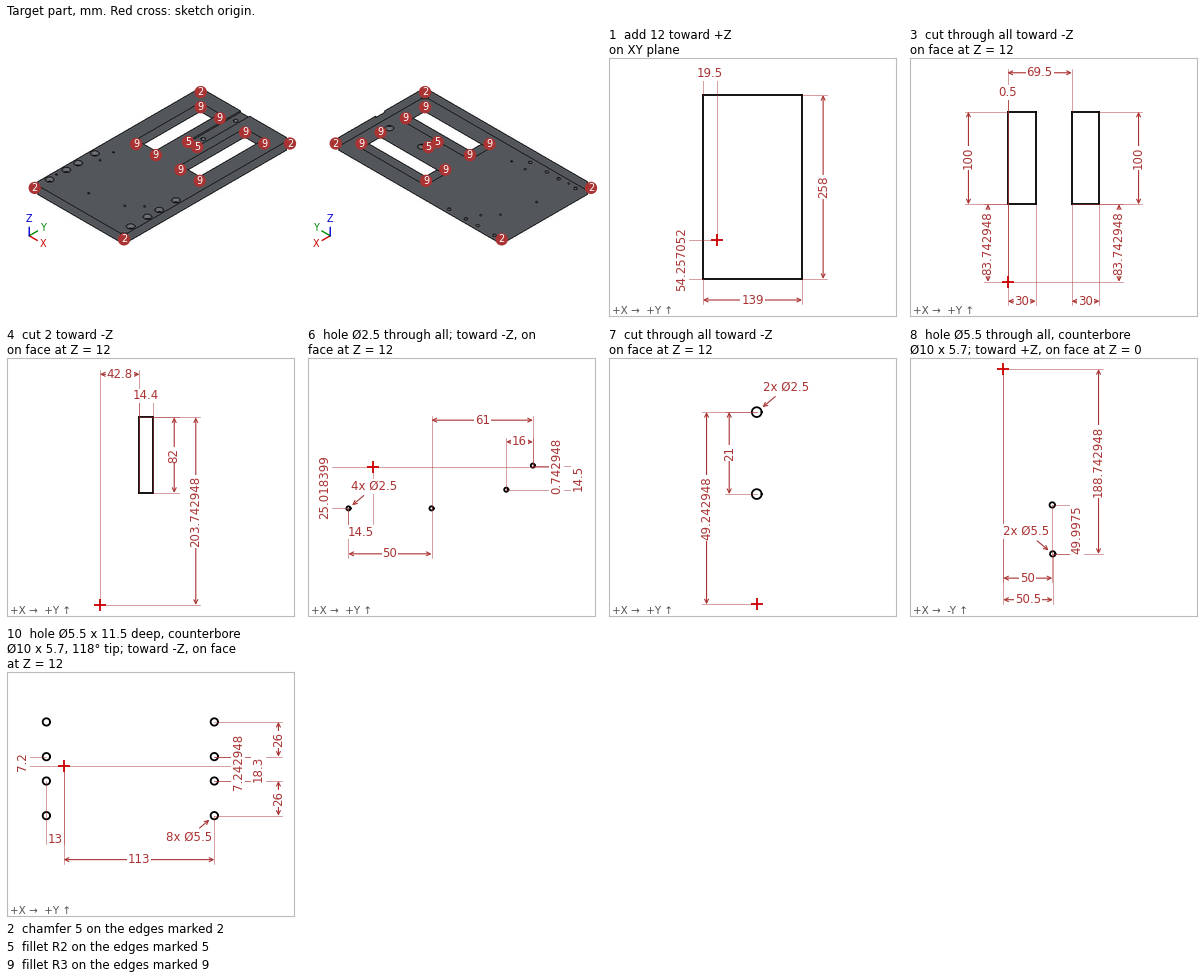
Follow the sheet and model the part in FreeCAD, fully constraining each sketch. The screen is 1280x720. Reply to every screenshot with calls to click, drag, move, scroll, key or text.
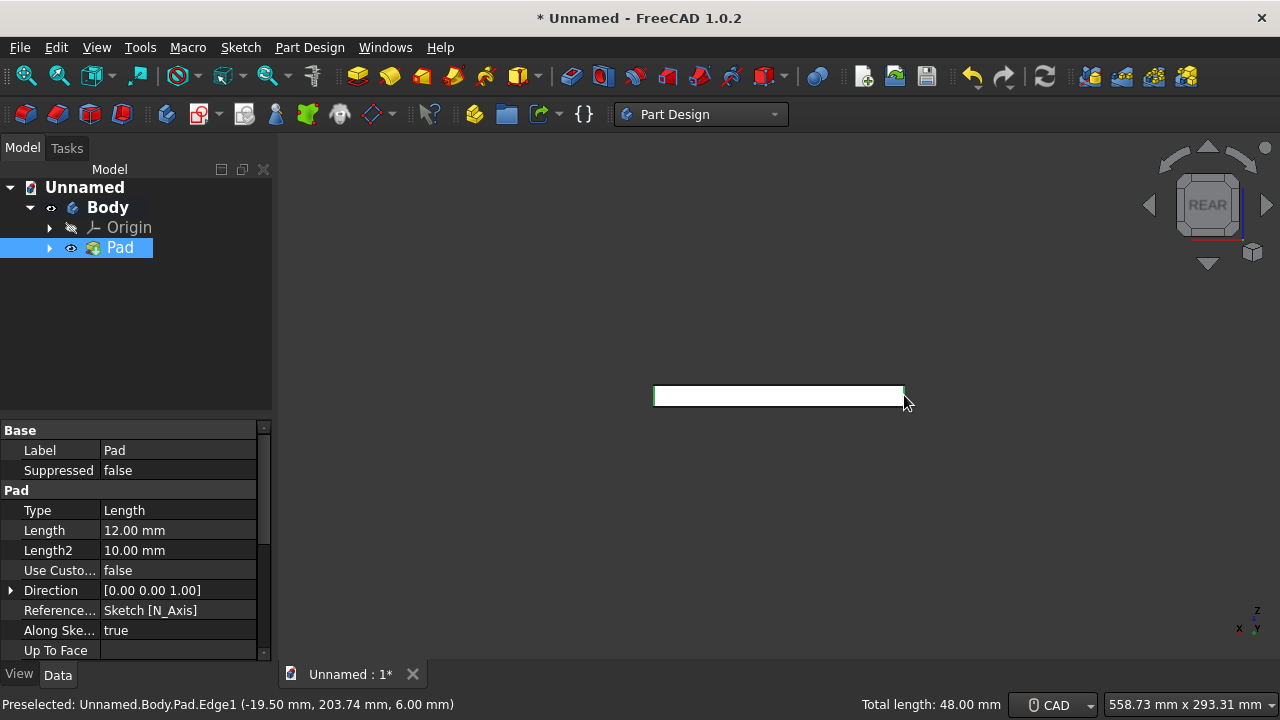
click(58, 114)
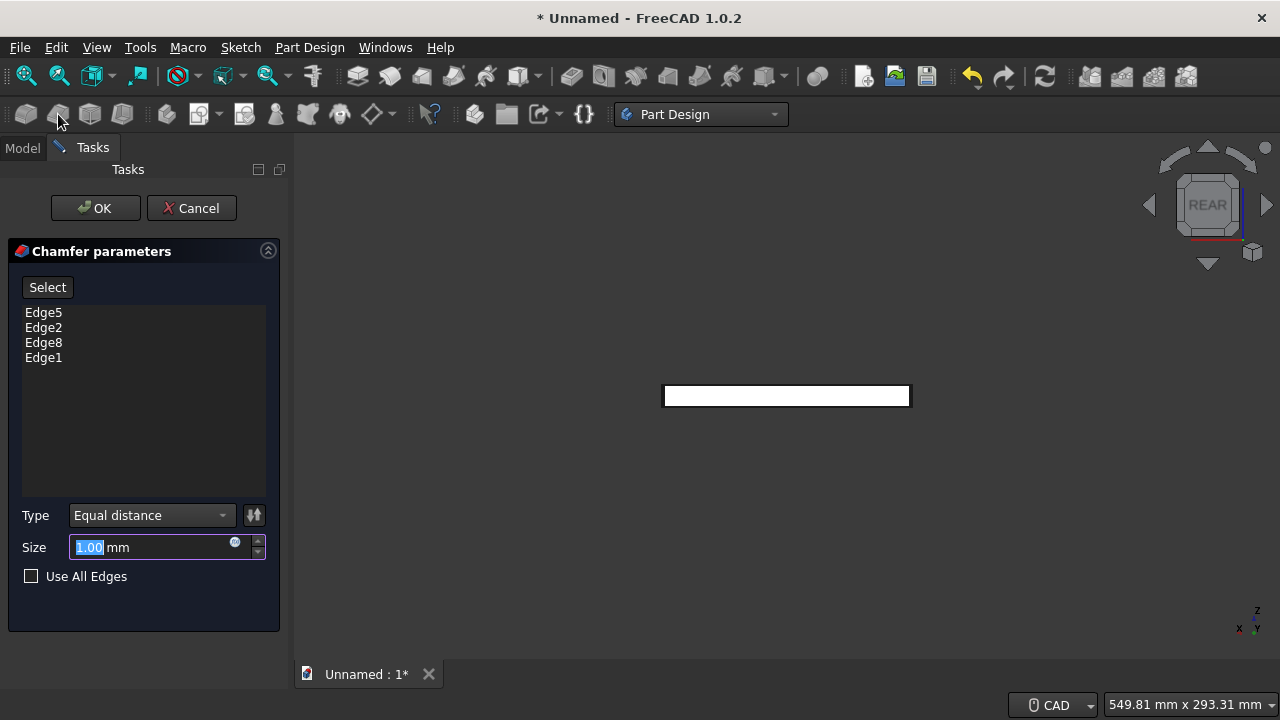
text(5)
key(Tab)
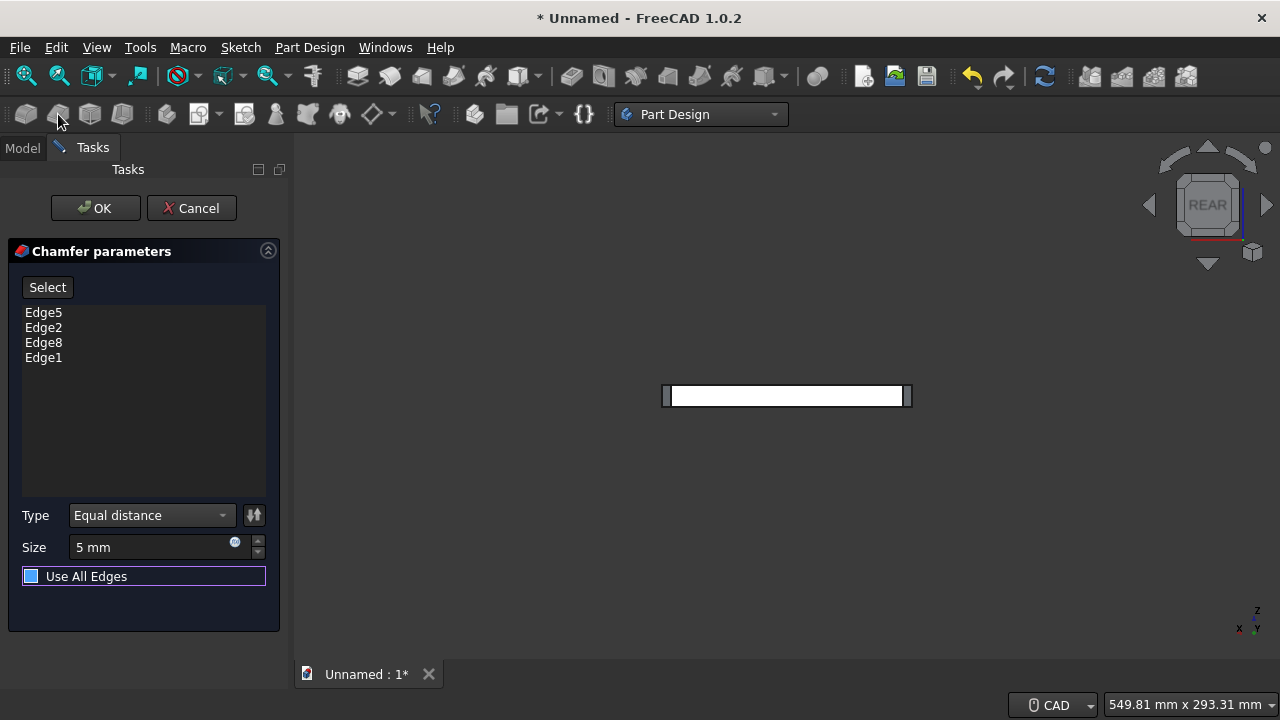
click(96, 208)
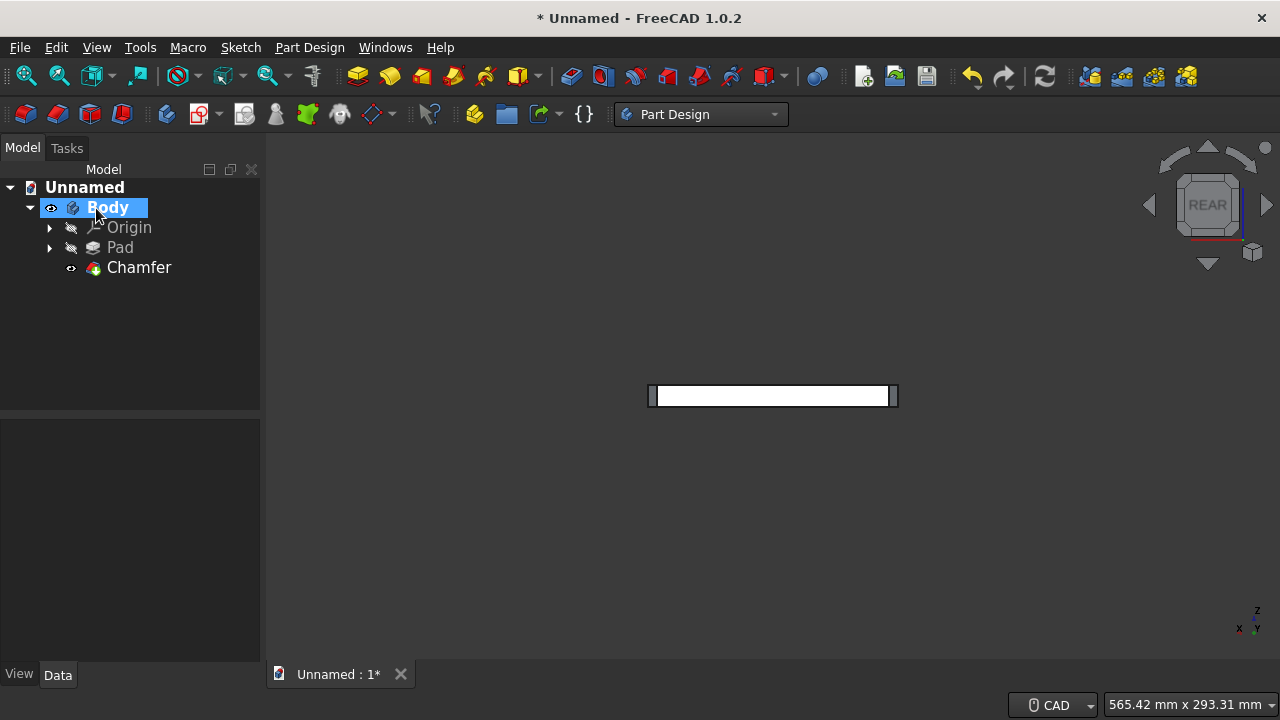
key(v)
key(f)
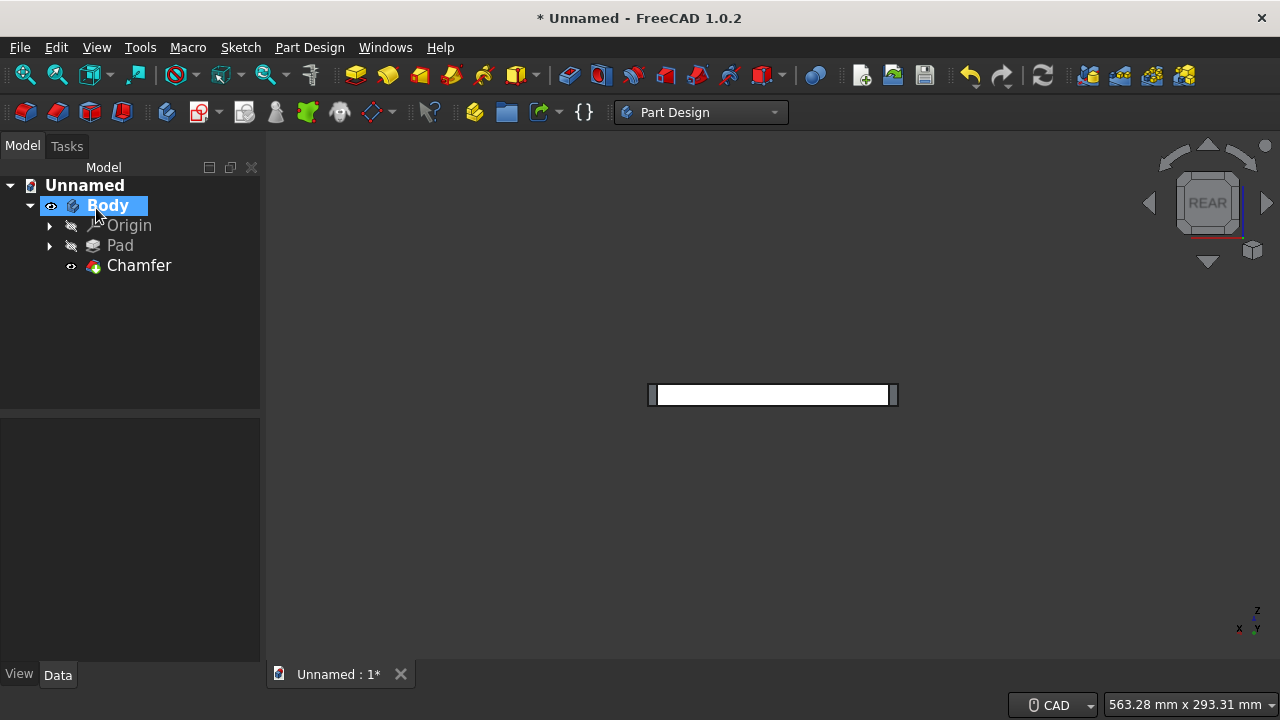
key(0)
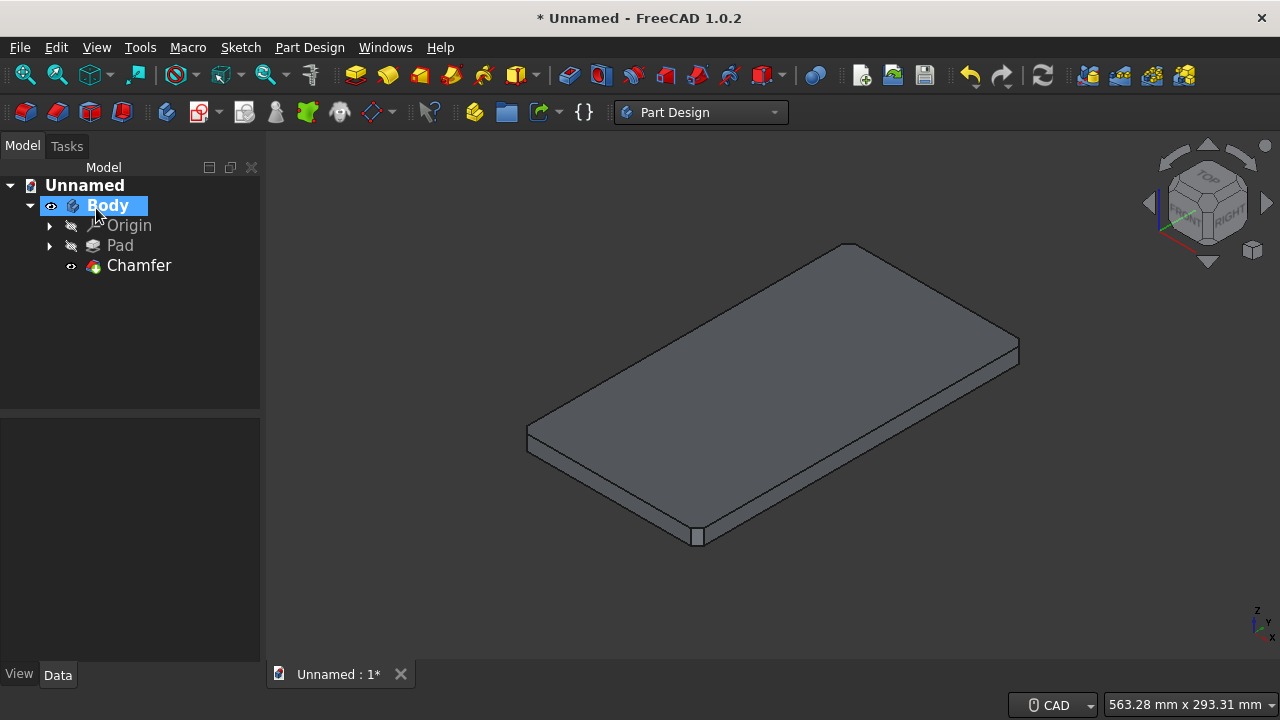
click(820, 358)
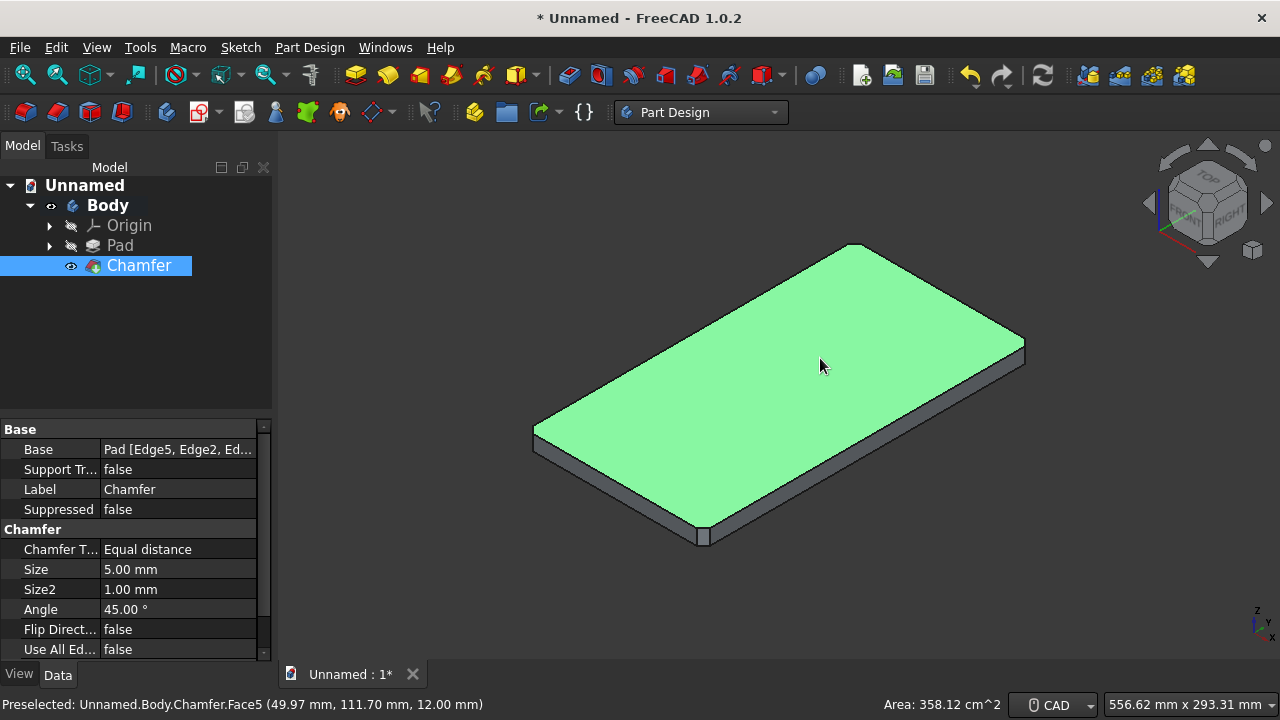
click(200, 112)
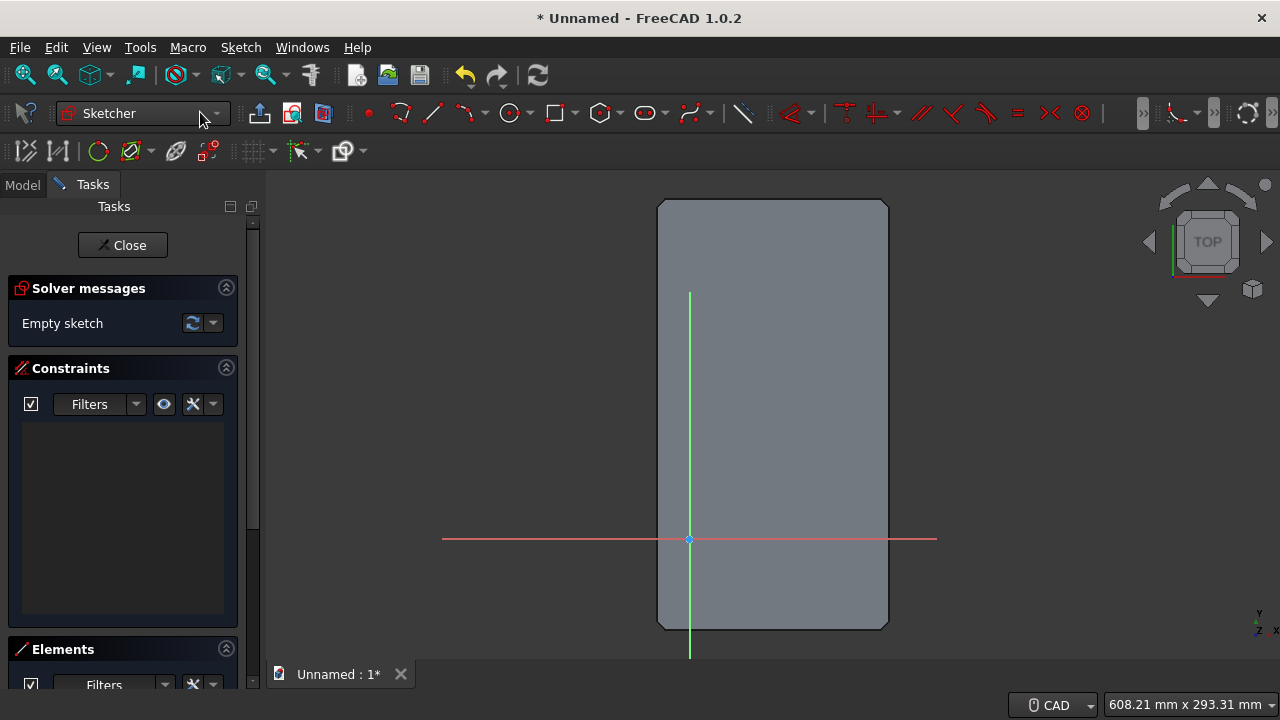
click(556, 114)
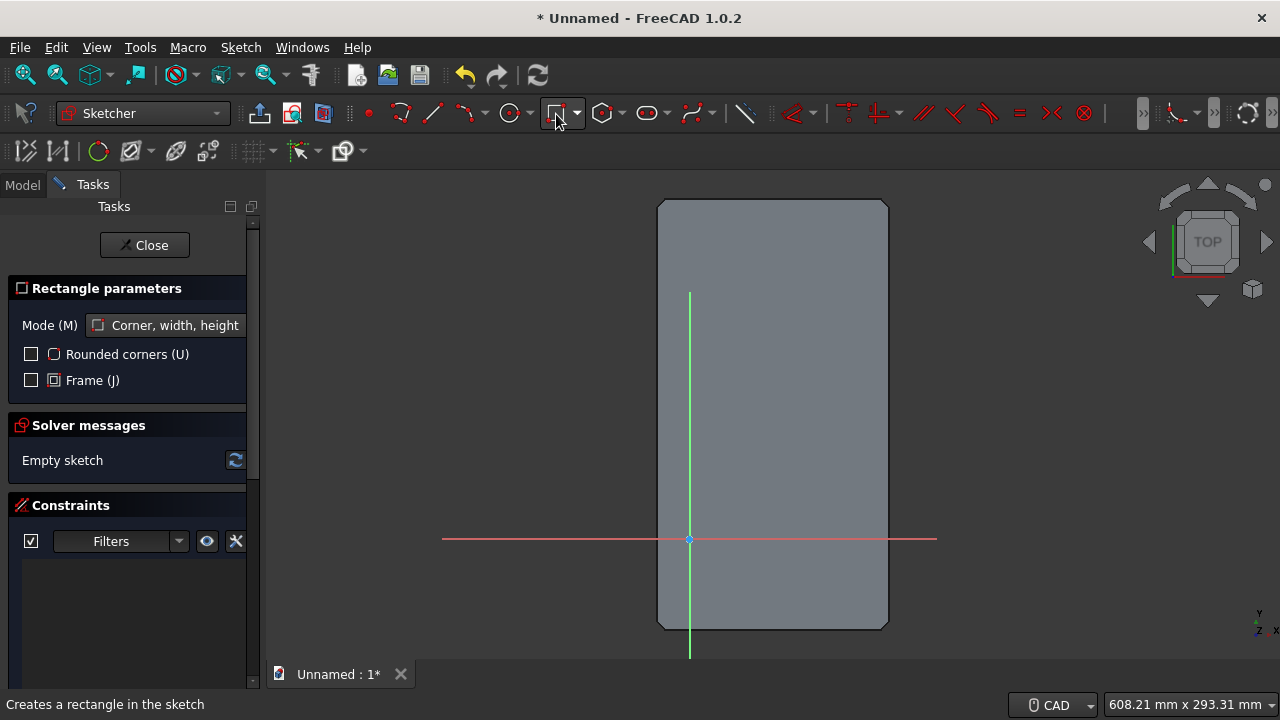
click(806, 233)
move(856, 399)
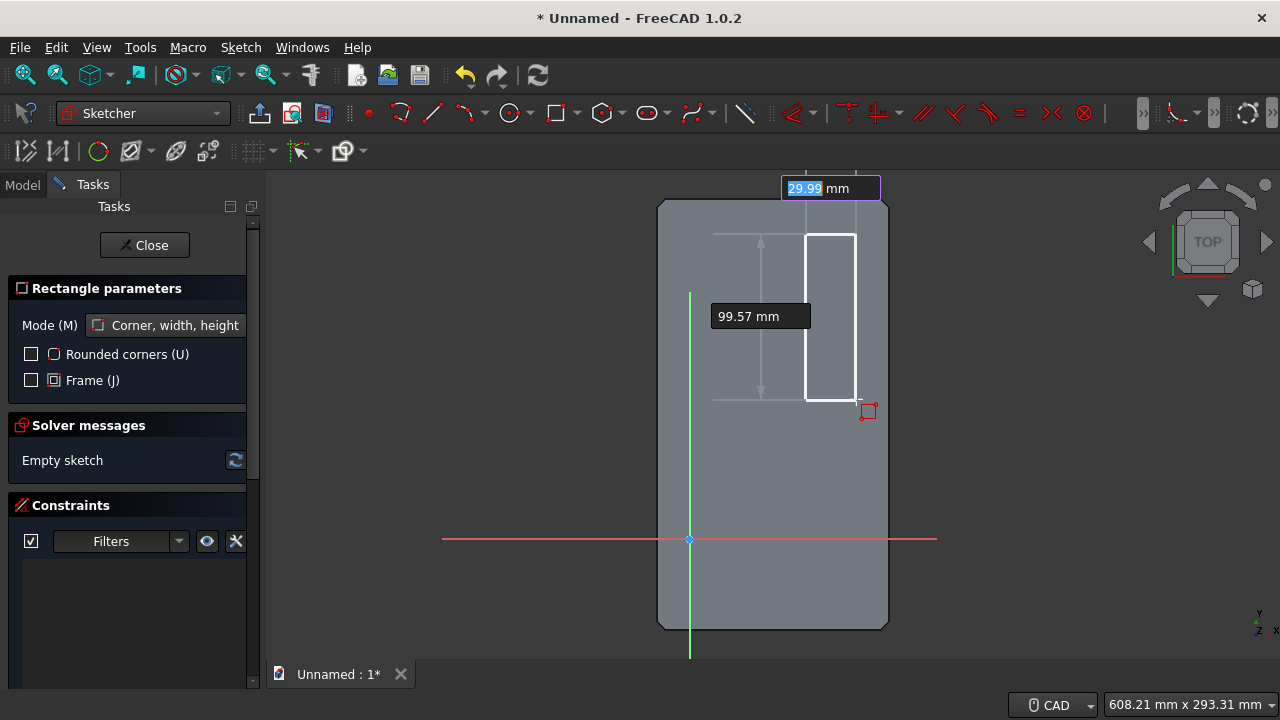
text(30)
key(Tab)
text(100)
key(Return)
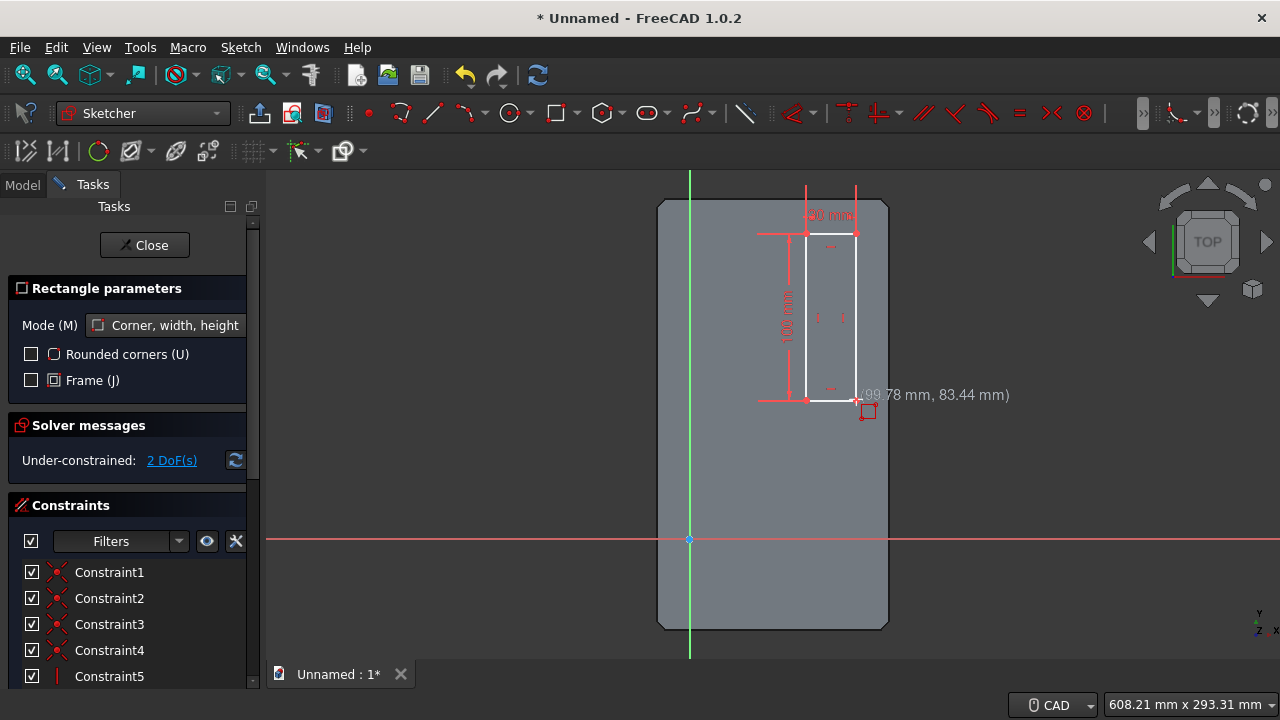
scroll(690, 233, up, 15)